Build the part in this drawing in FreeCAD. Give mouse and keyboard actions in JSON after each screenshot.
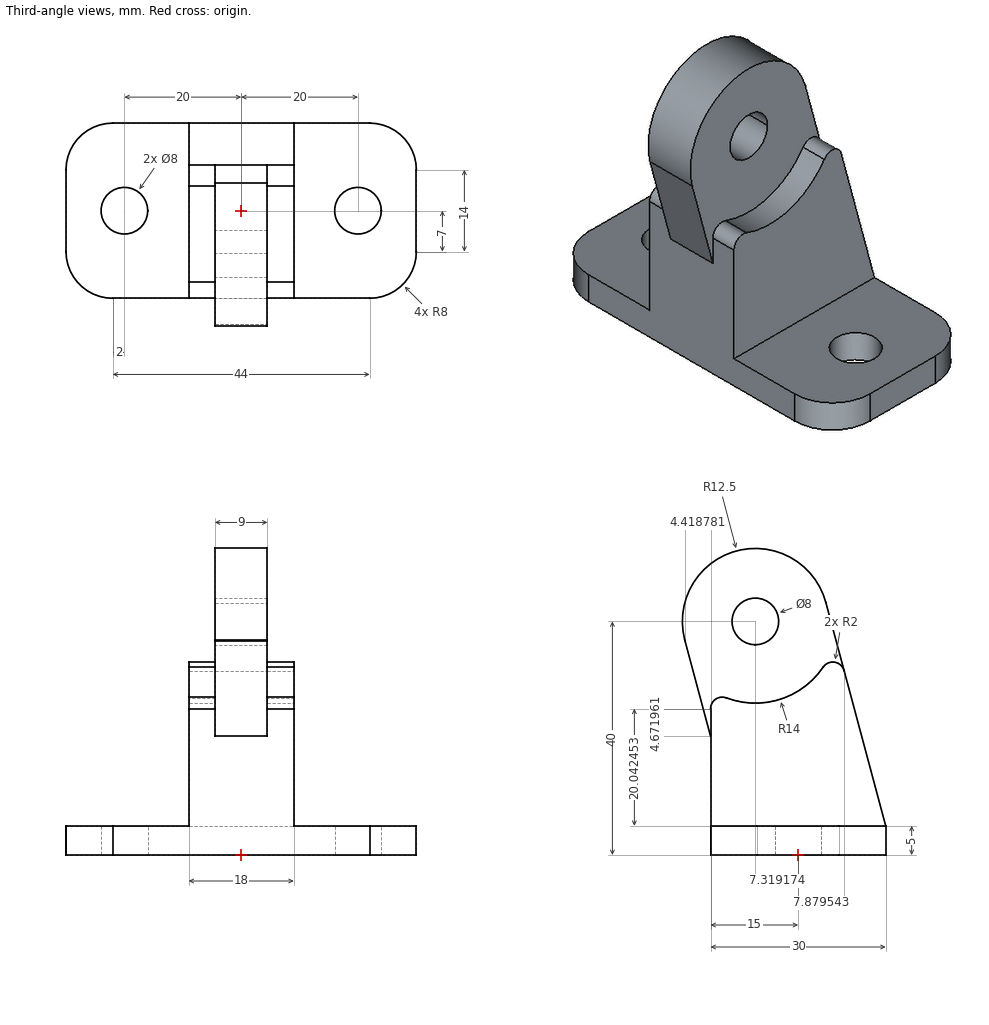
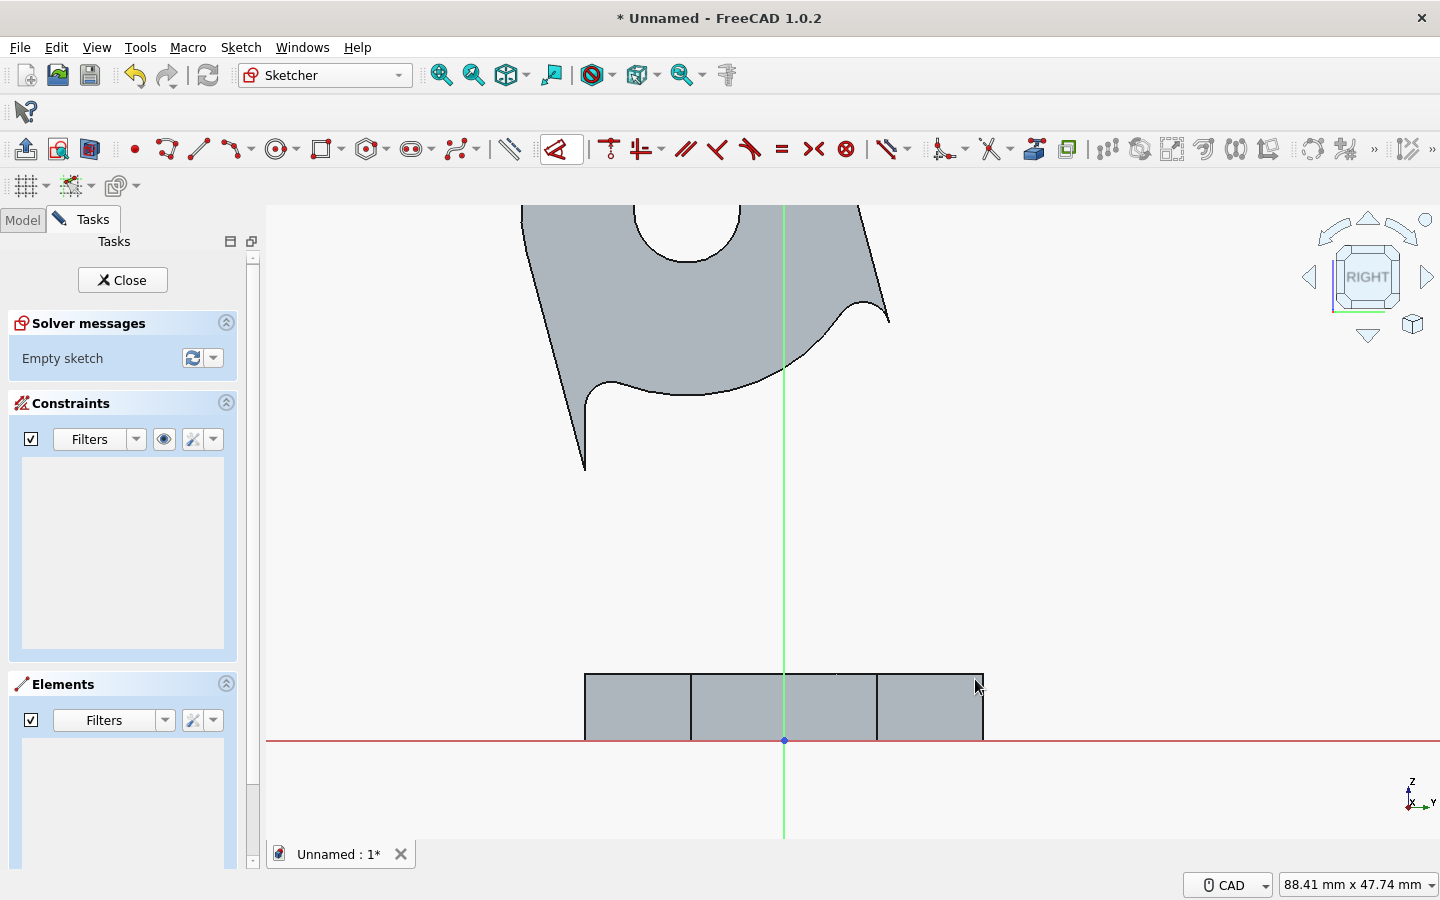
{"action": "left_click", "coordinate": [168, 150]}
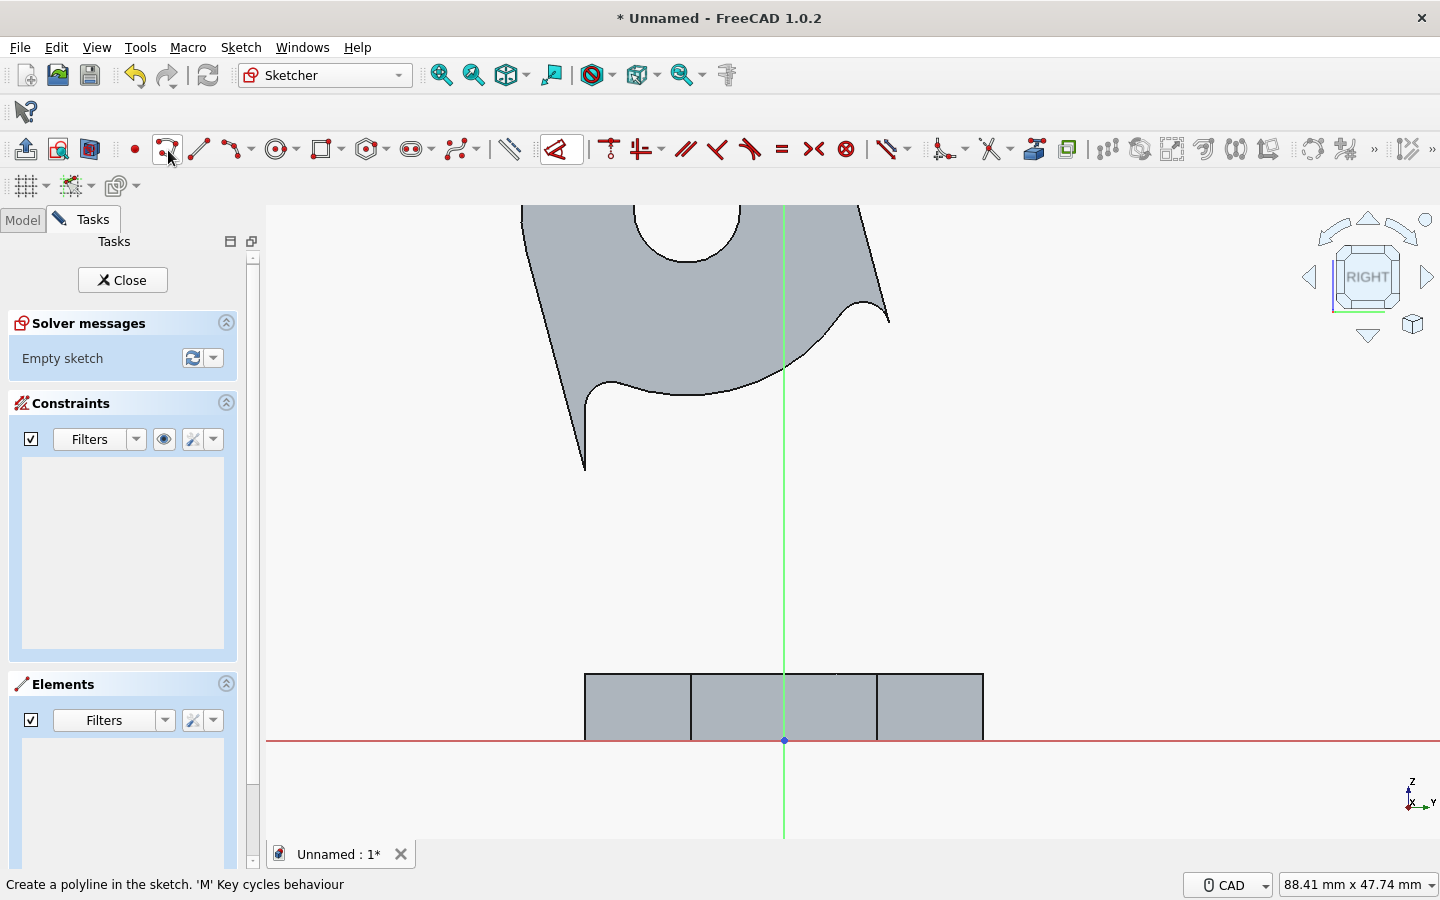
{"action": "left_click", "coordinate": [585, 408]}
{"action": "left_click", "coordinate": [585, 674]}
{"action": "left_click", "coordinate": [983, 674]}
{"action": "left_click", "coordinate": [889, 322]}
{"action": "right_click", "coordinate": [889, 322]}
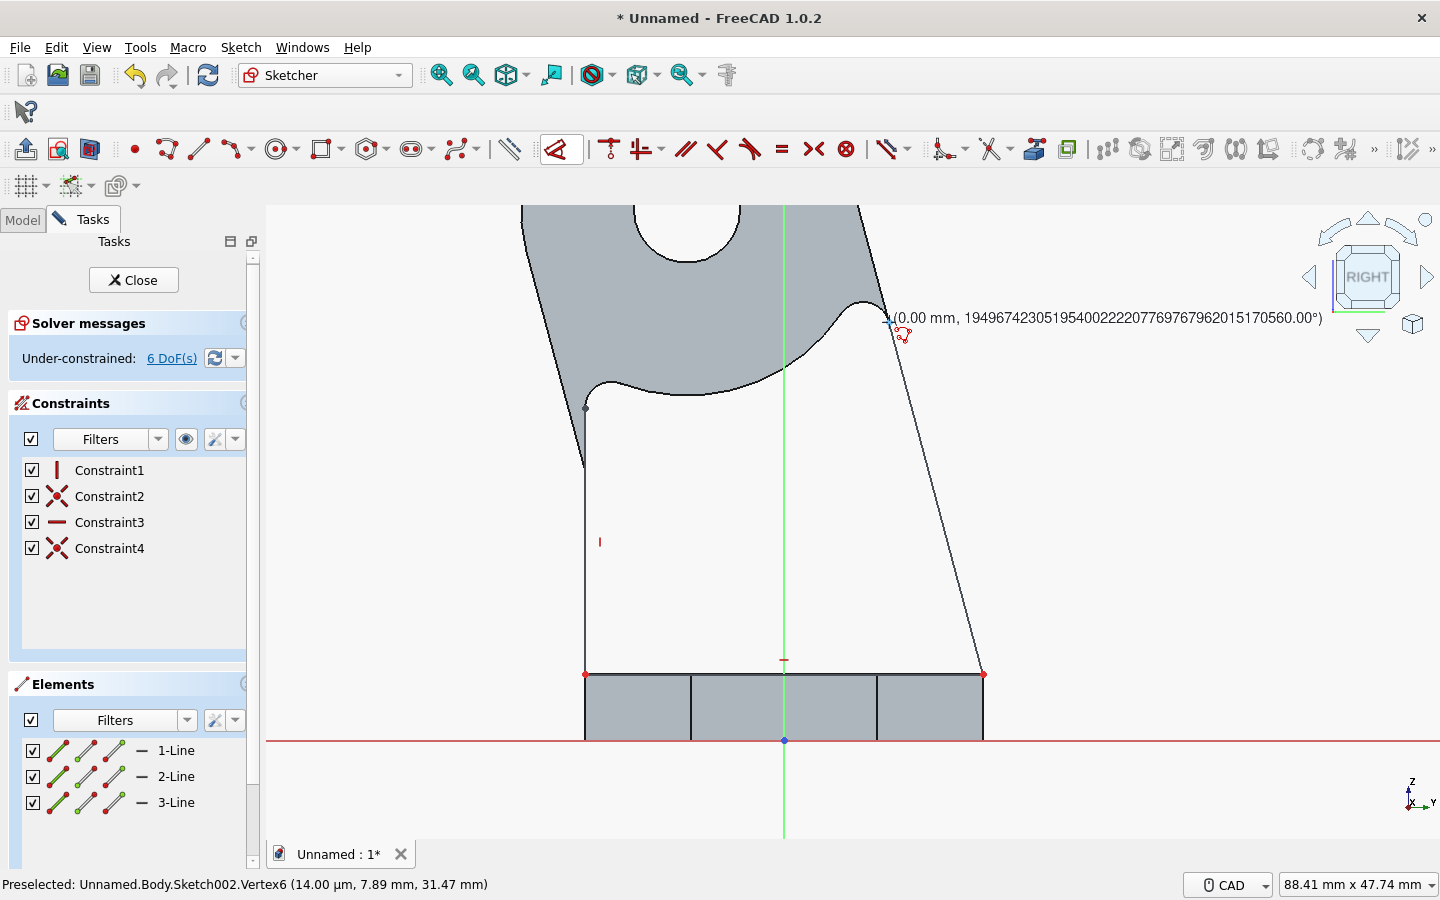
{"action": "left_click", "coordinate": [232, 150]}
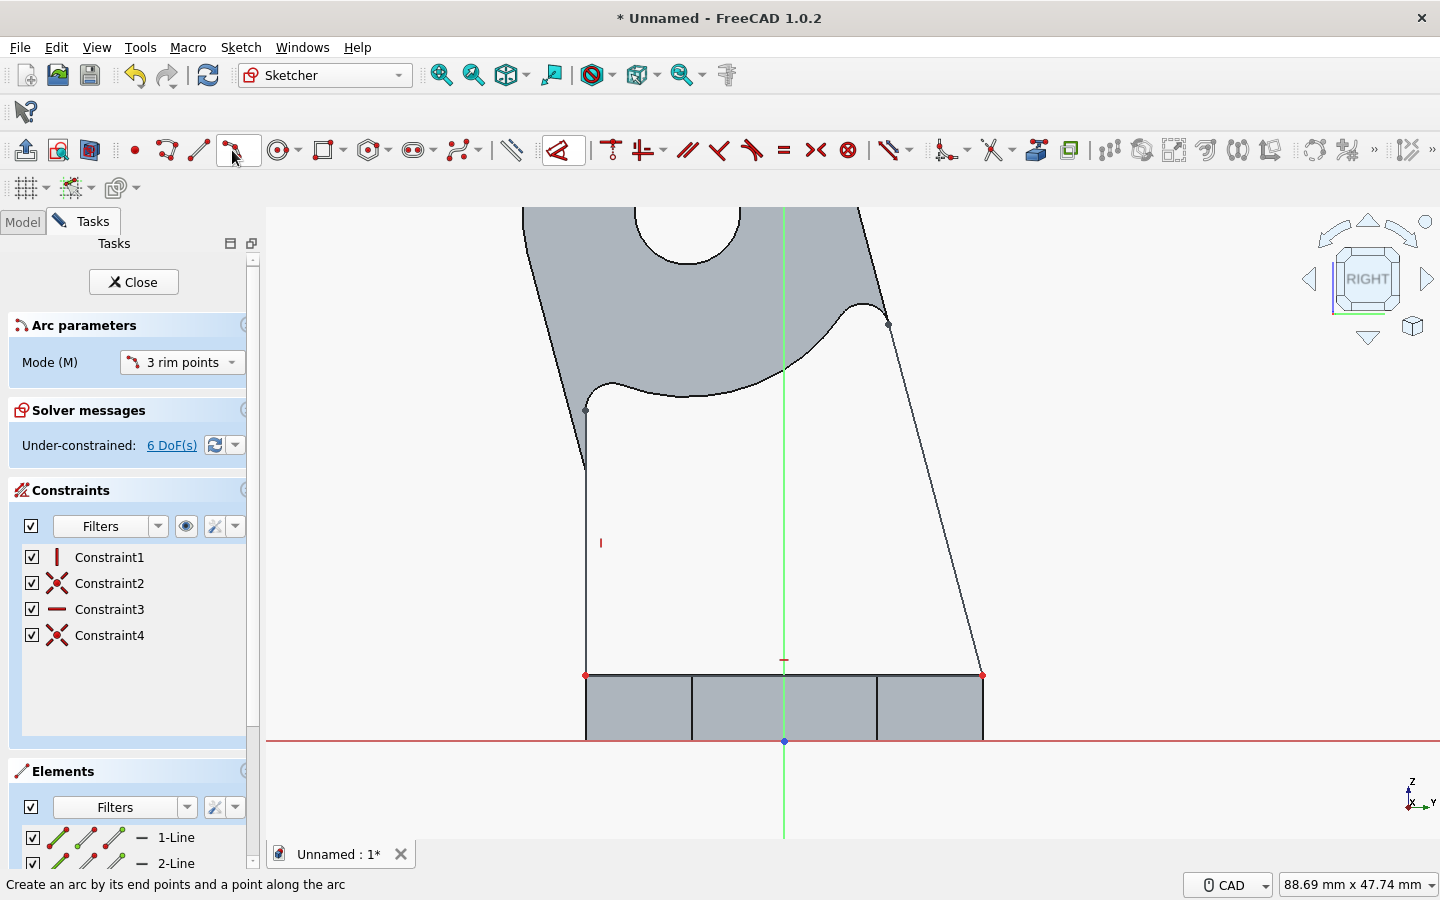
{"action": "left_click", "coordinate": [889, 325]}
{"action": "left_click", "coordinate": [841, 315]}
{"action": "left_click", "coordinate": [868, 304]}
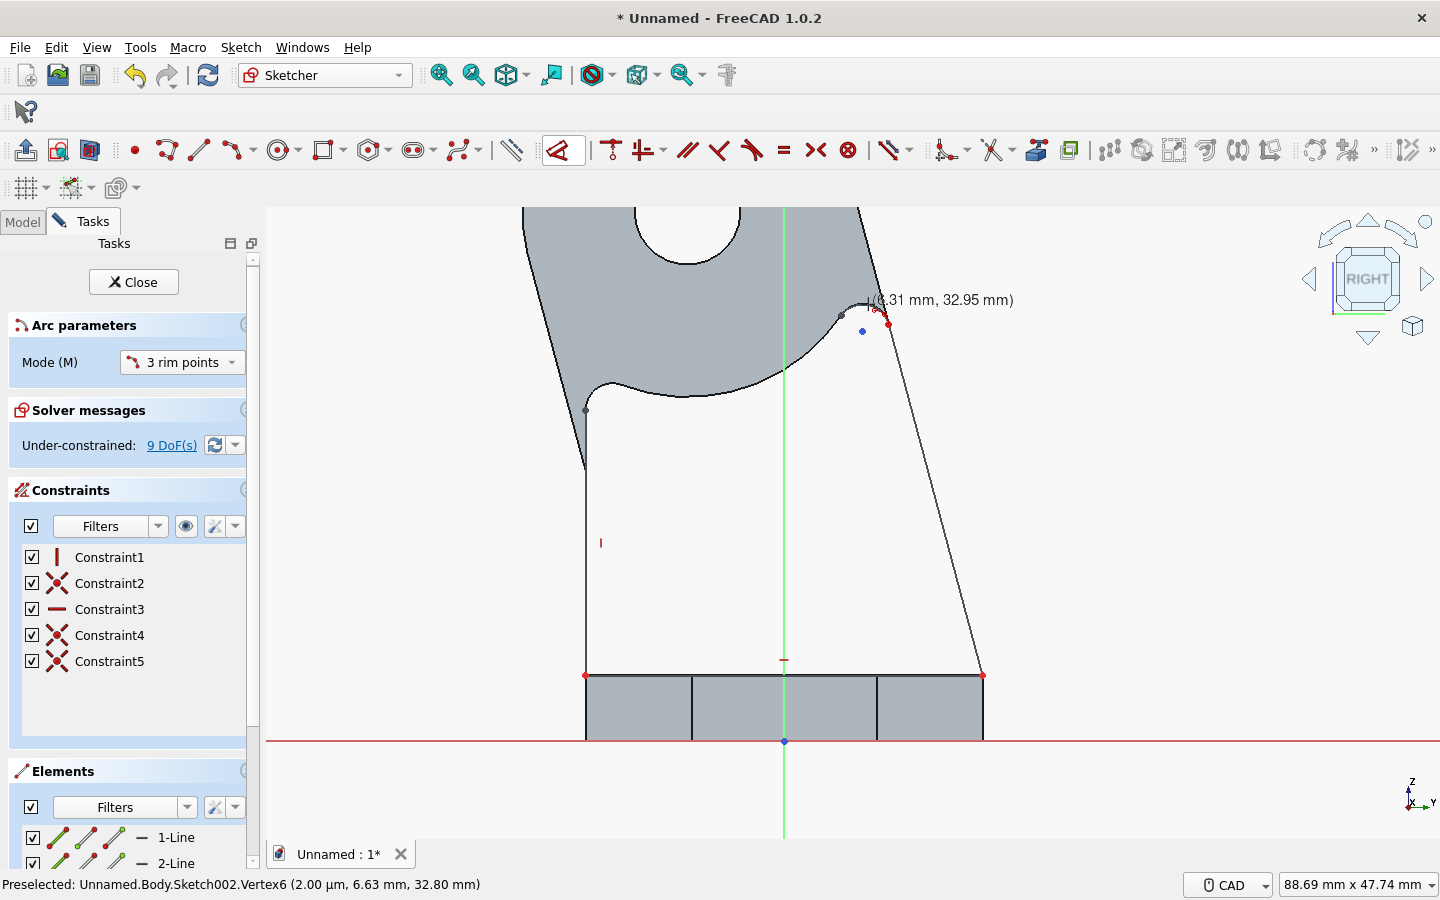
{"action": "left_click", "coordinate": [841, 316]}
{"action": "left_click", "coordinate": [622, 385]}
{"action": "left_click", "coordinate": [744, 388]}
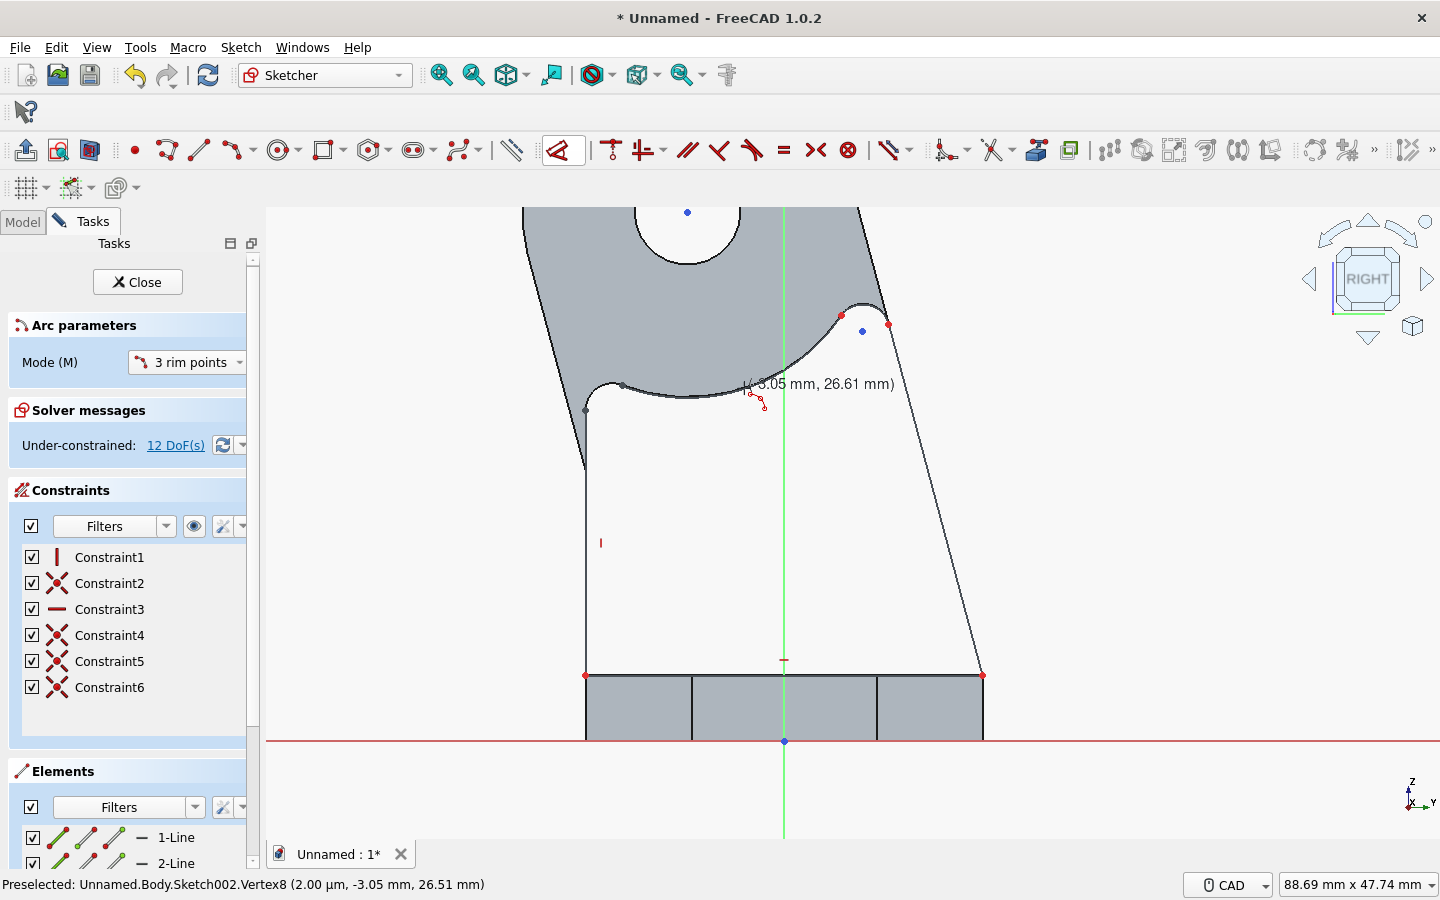
{"action": "left_click", "coordinate": [622, 386]}
{"action": "left_click", "coordinate": [586, 410]}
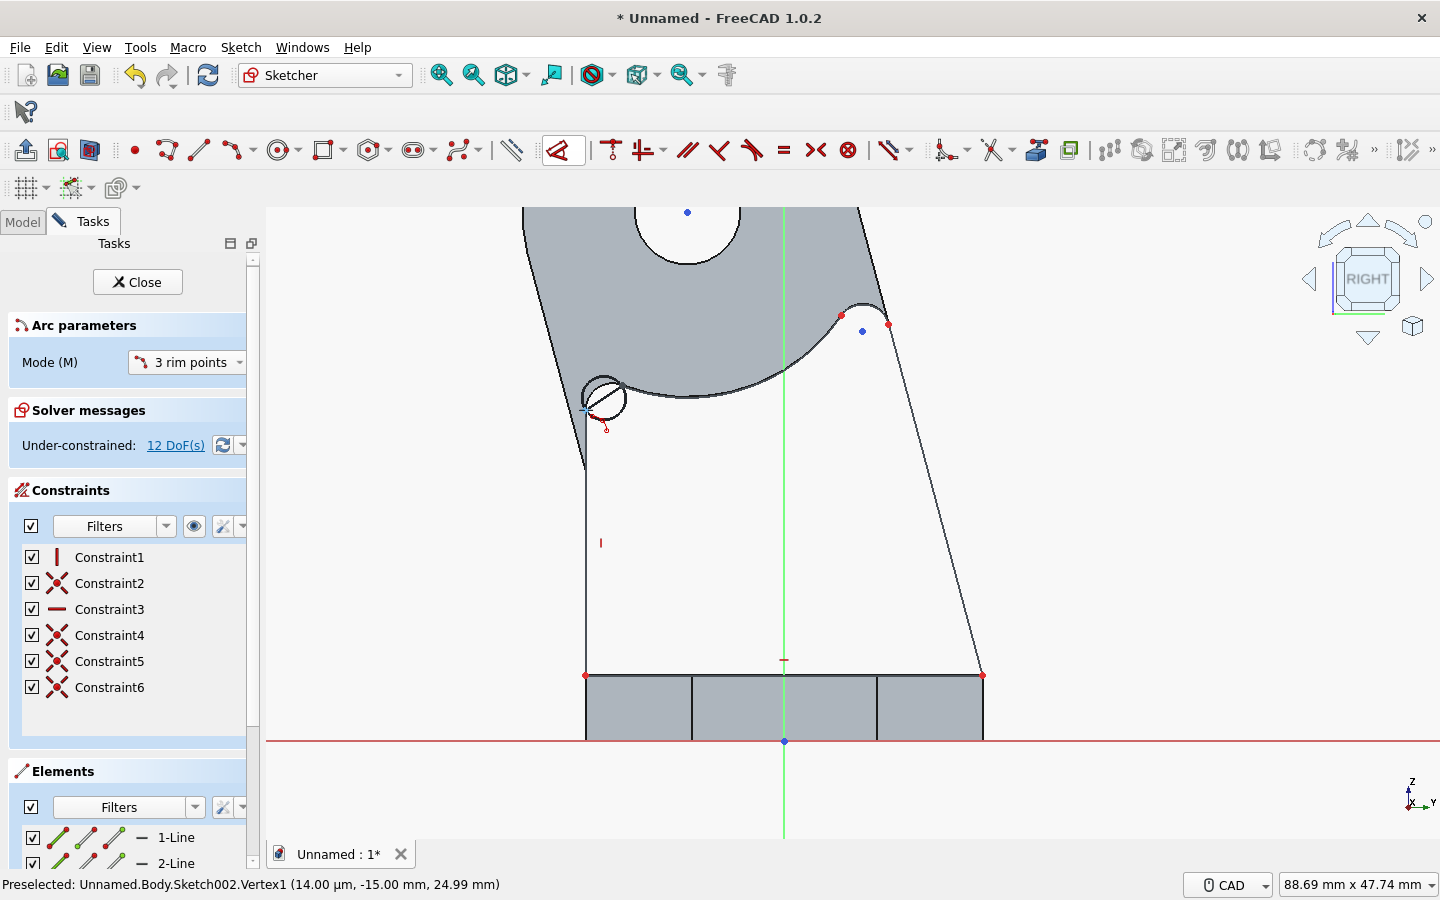
{"action": "scroll", "coordinate": [597, 388], "scroll_direction": "up", "scroll_amount": 2}